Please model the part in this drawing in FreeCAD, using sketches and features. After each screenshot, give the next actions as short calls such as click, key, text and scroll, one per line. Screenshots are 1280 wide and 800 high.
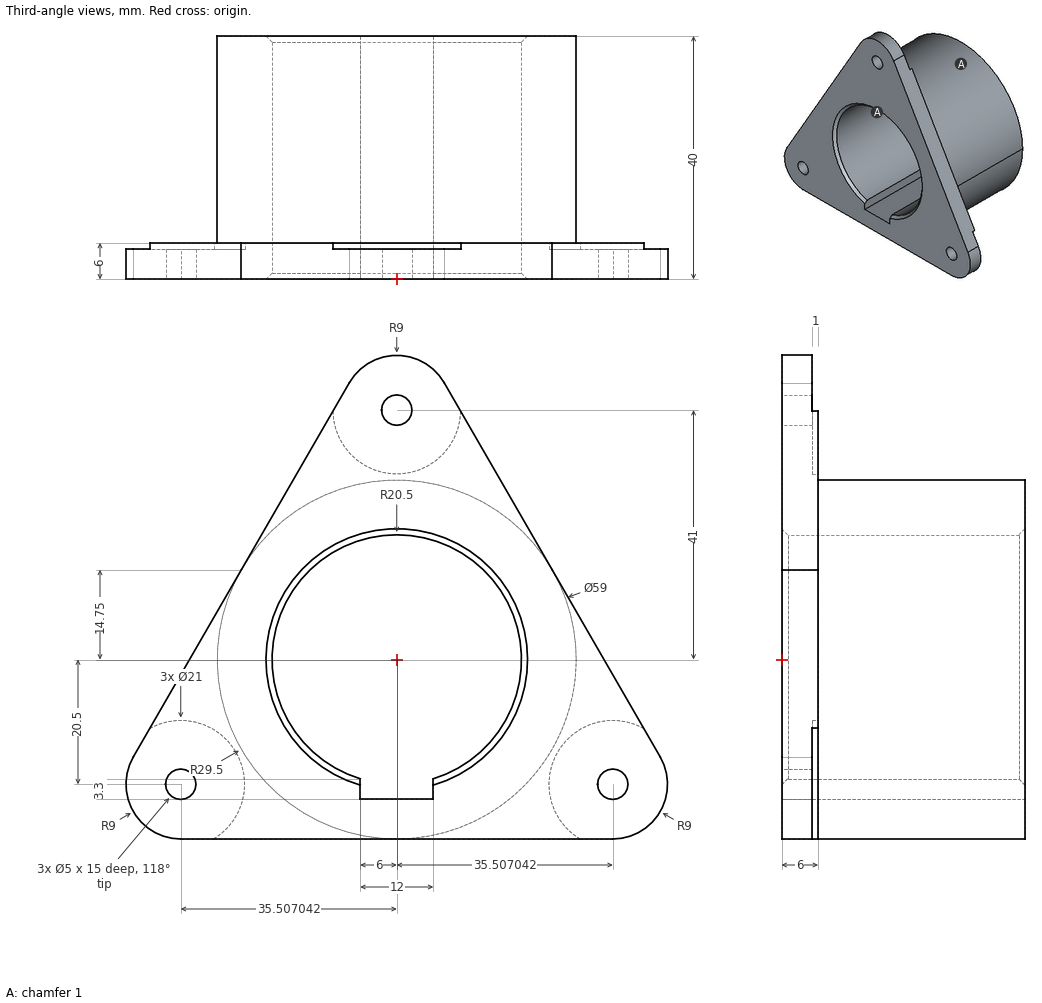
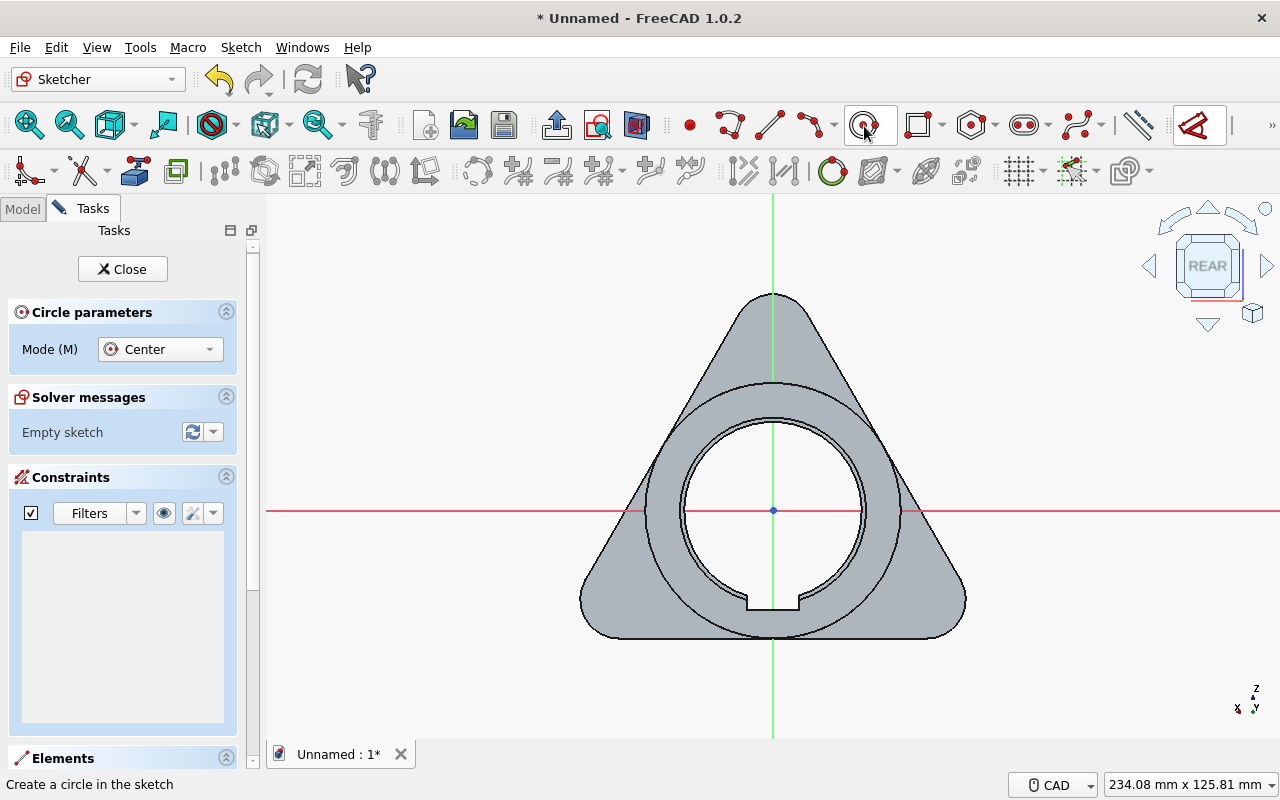
scroll(927, 600, up, 4)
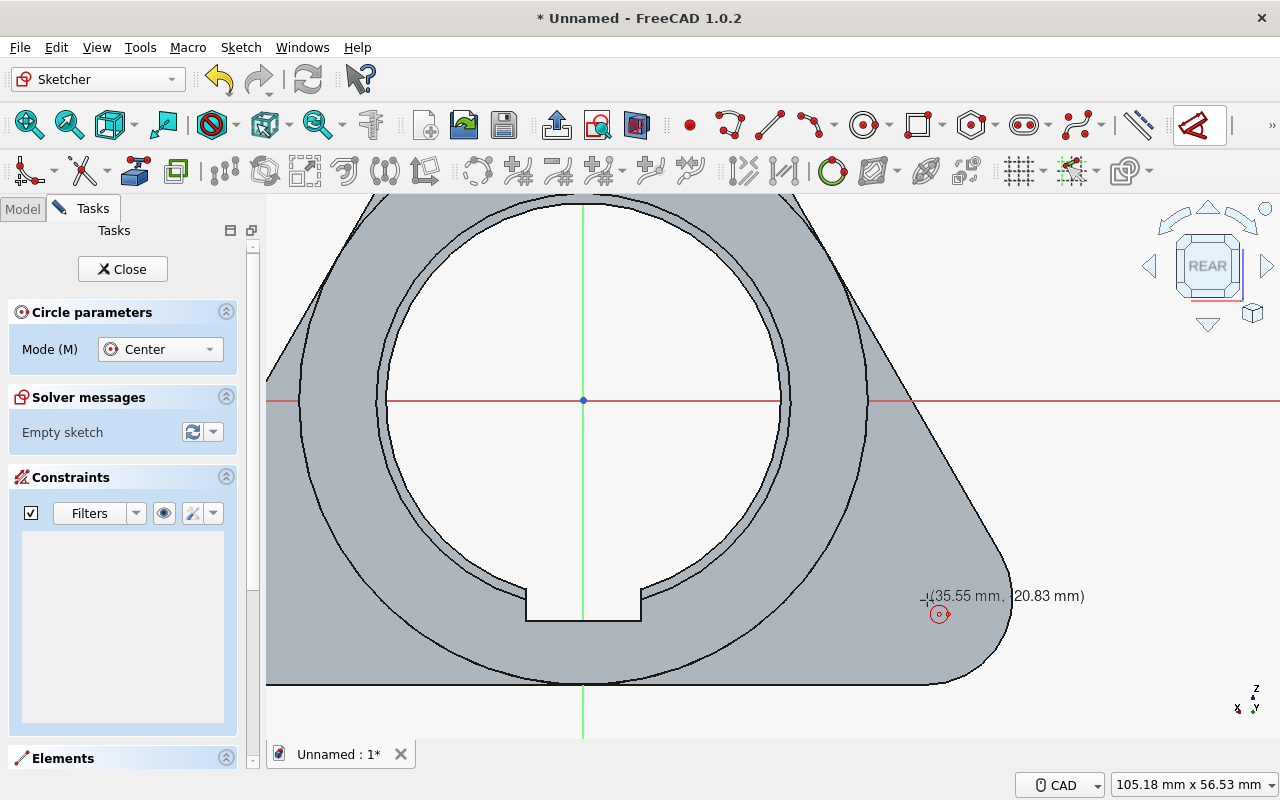
click(926, 598)
click(943, 581)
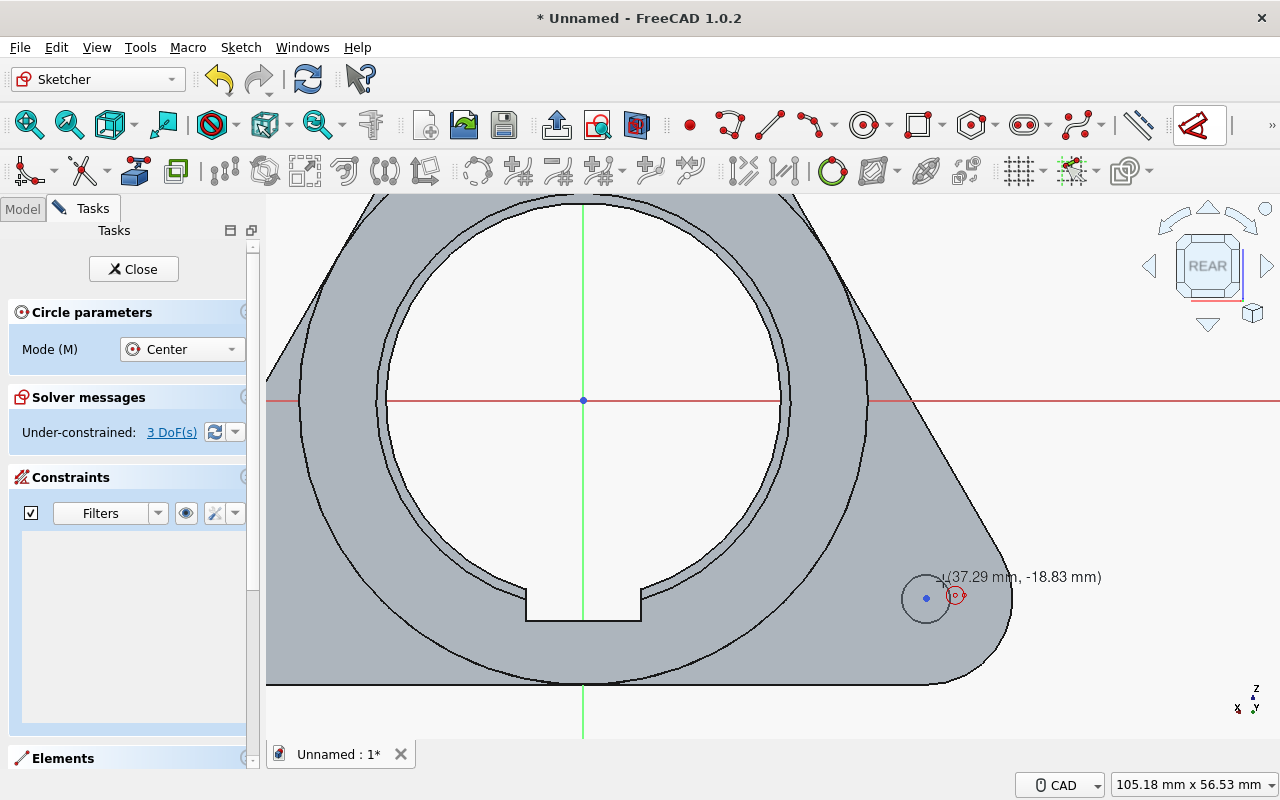
scroll(852, 667, down, 3)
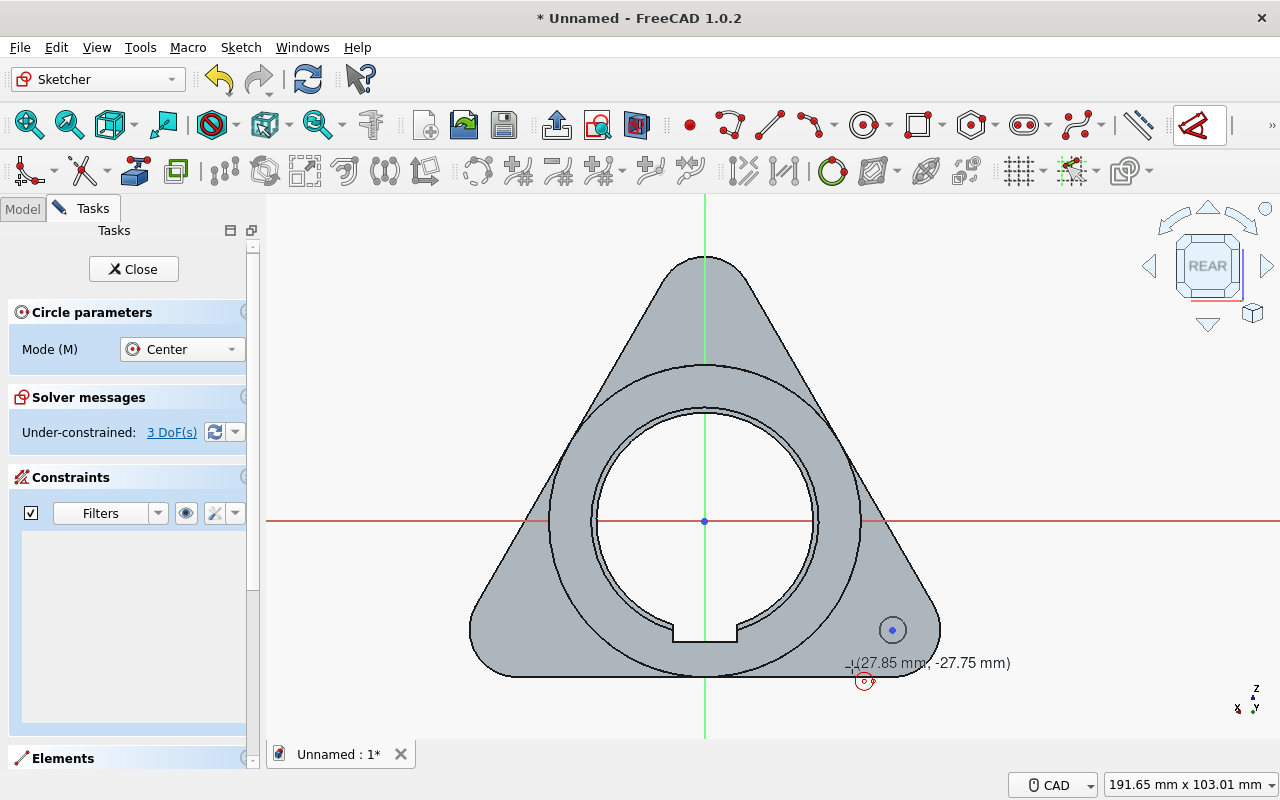
scroll(517, 630, up, 3)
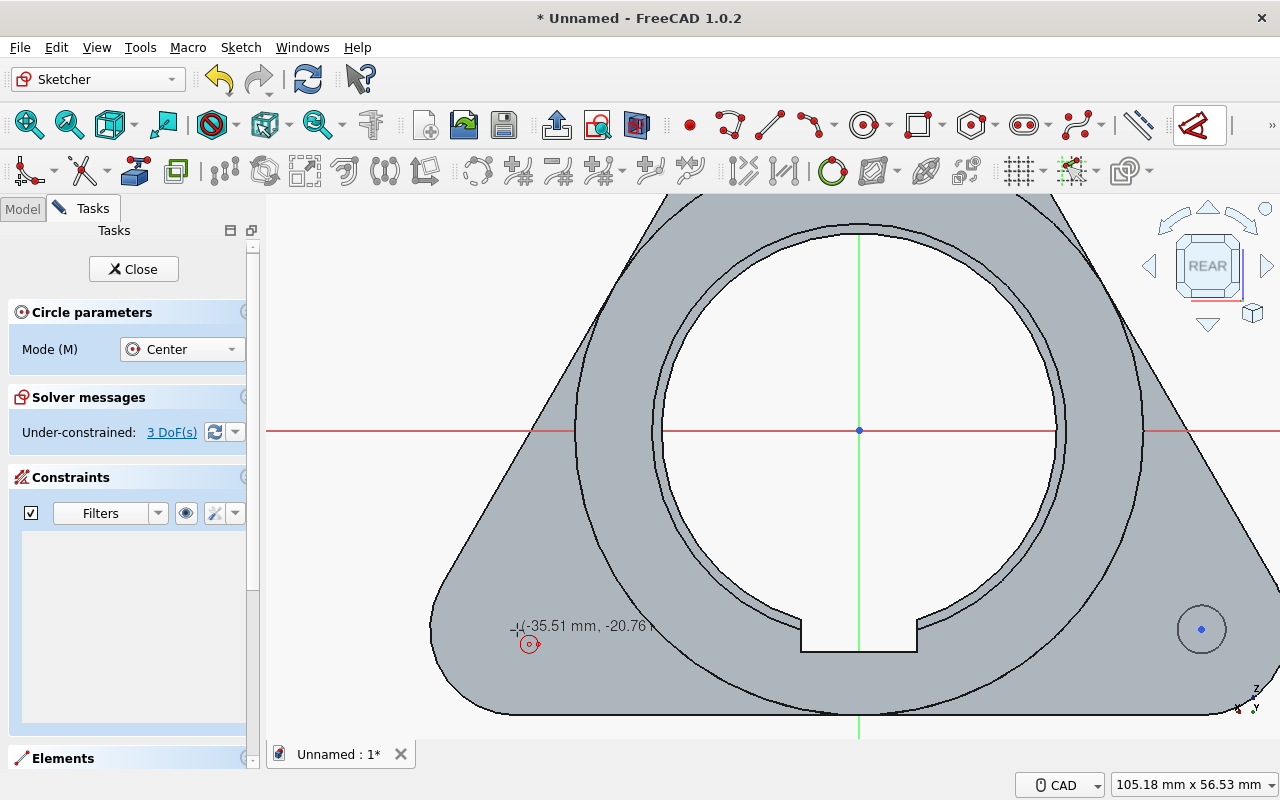
click(517, 629)
click(534, 612)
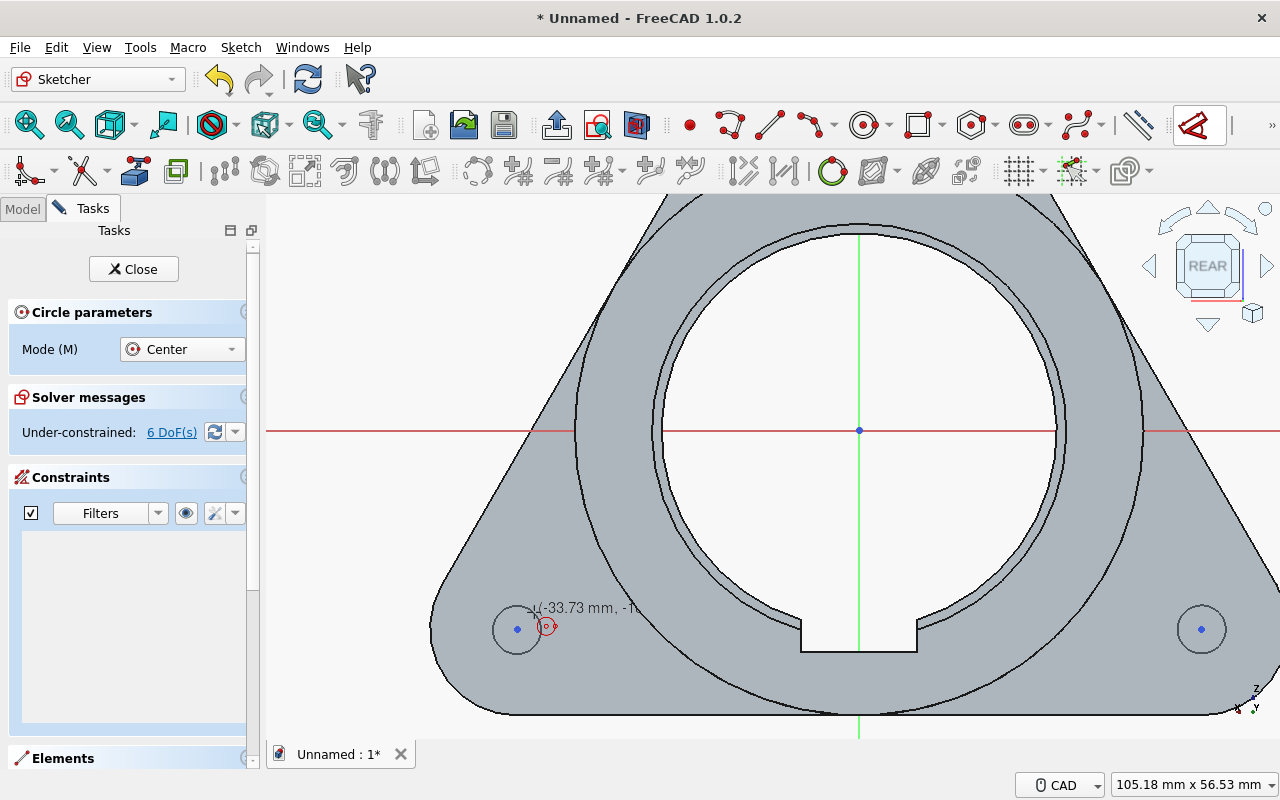
scroll(516, 630, down, 3)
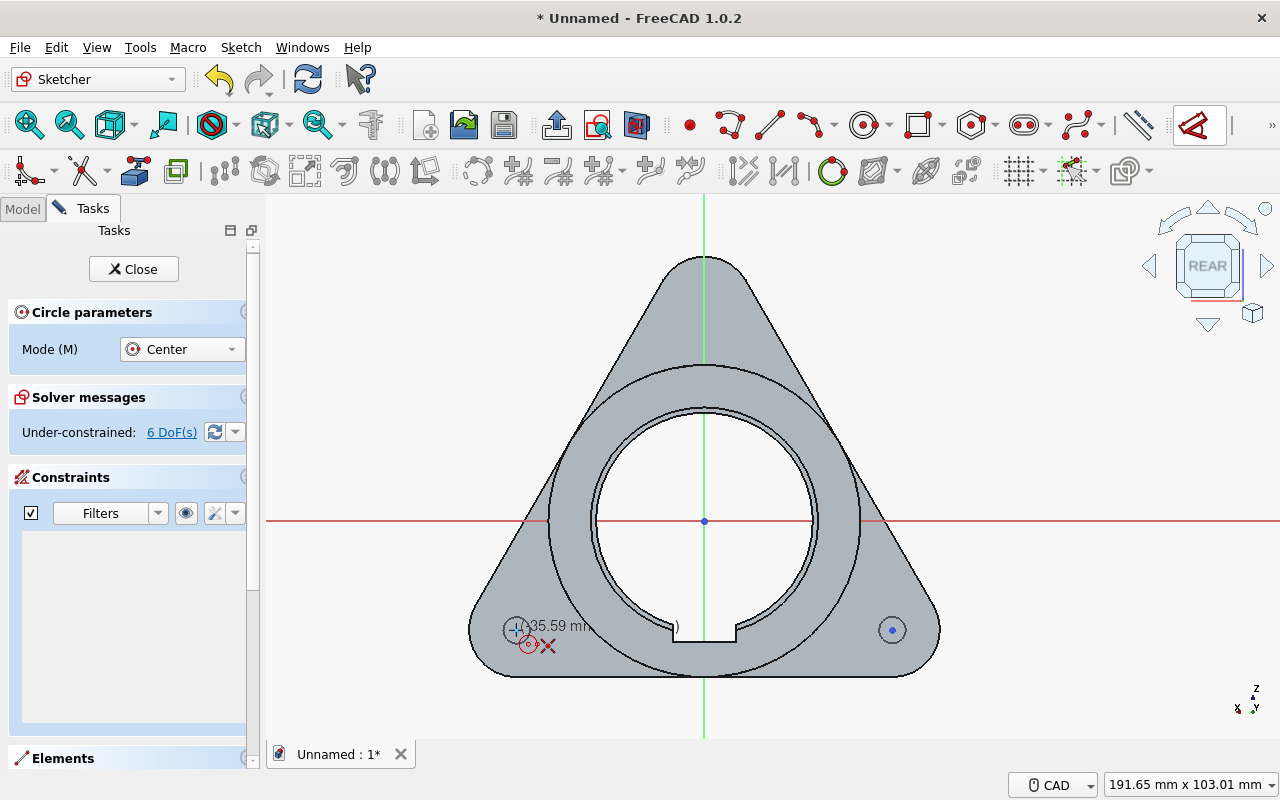
scroll(704, 304, up, 3)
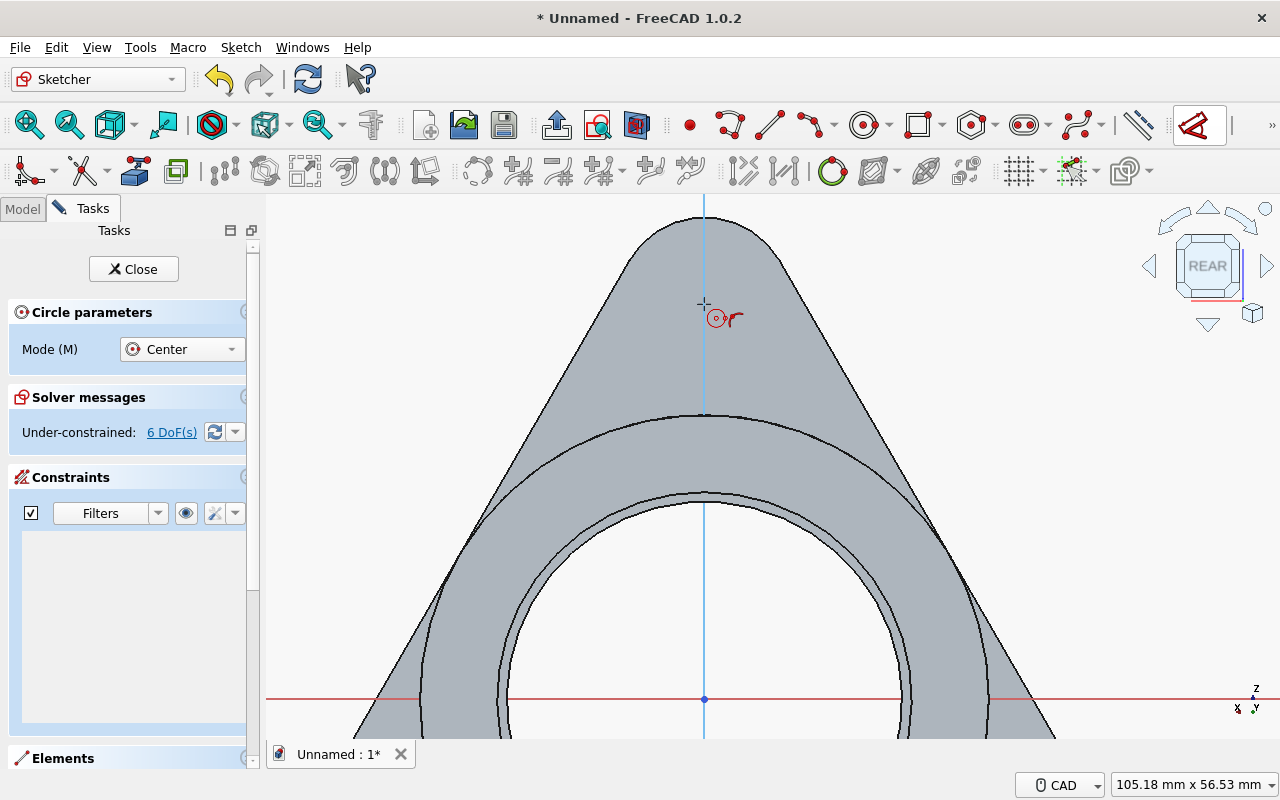
click(704, 304)
click(721, 287)
key(Escape)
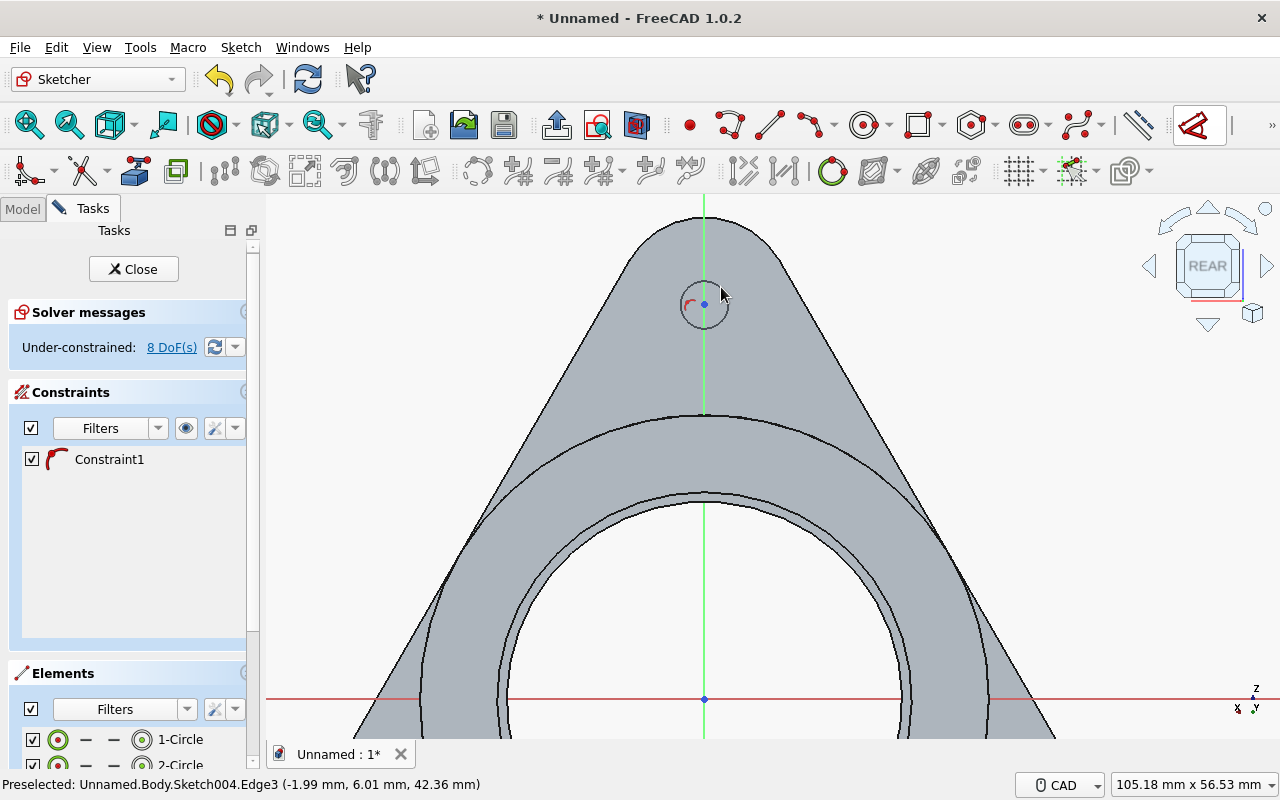
scroll(705, 303, down, 3)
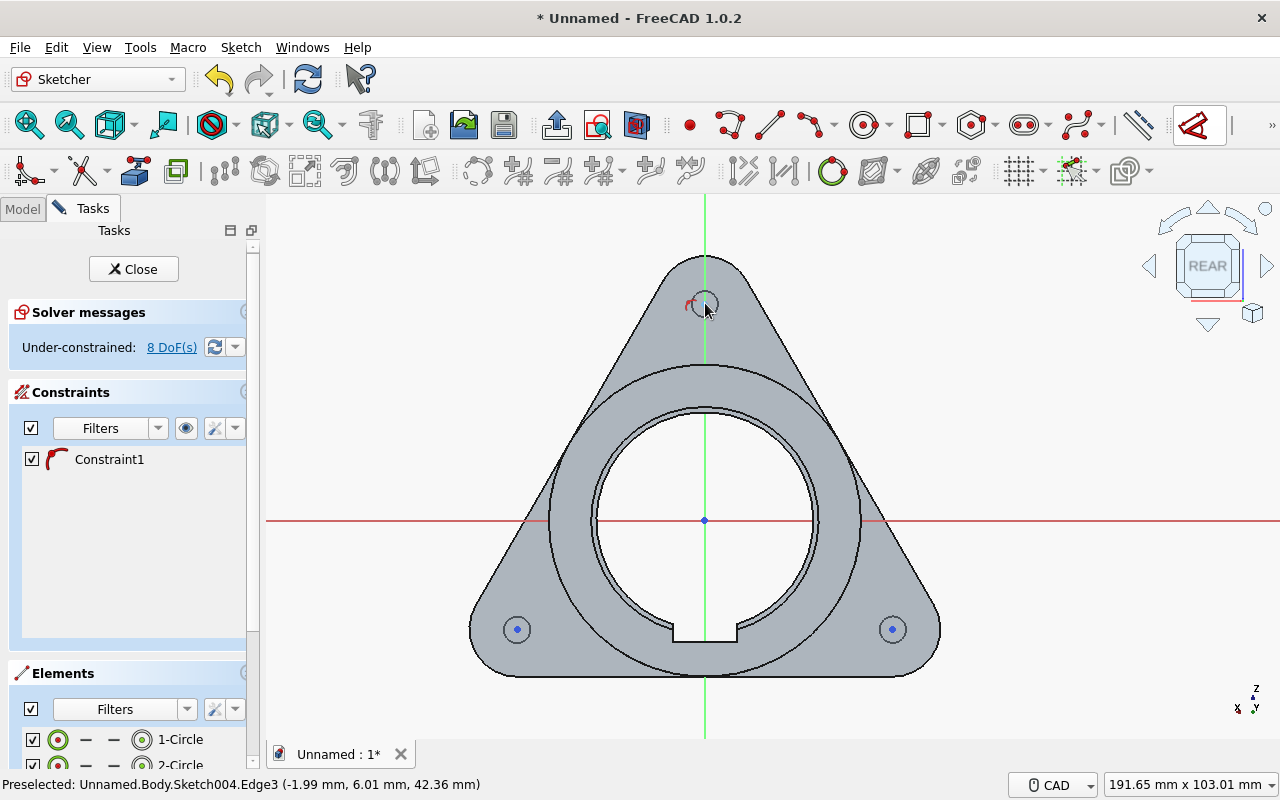
click(902, 620)